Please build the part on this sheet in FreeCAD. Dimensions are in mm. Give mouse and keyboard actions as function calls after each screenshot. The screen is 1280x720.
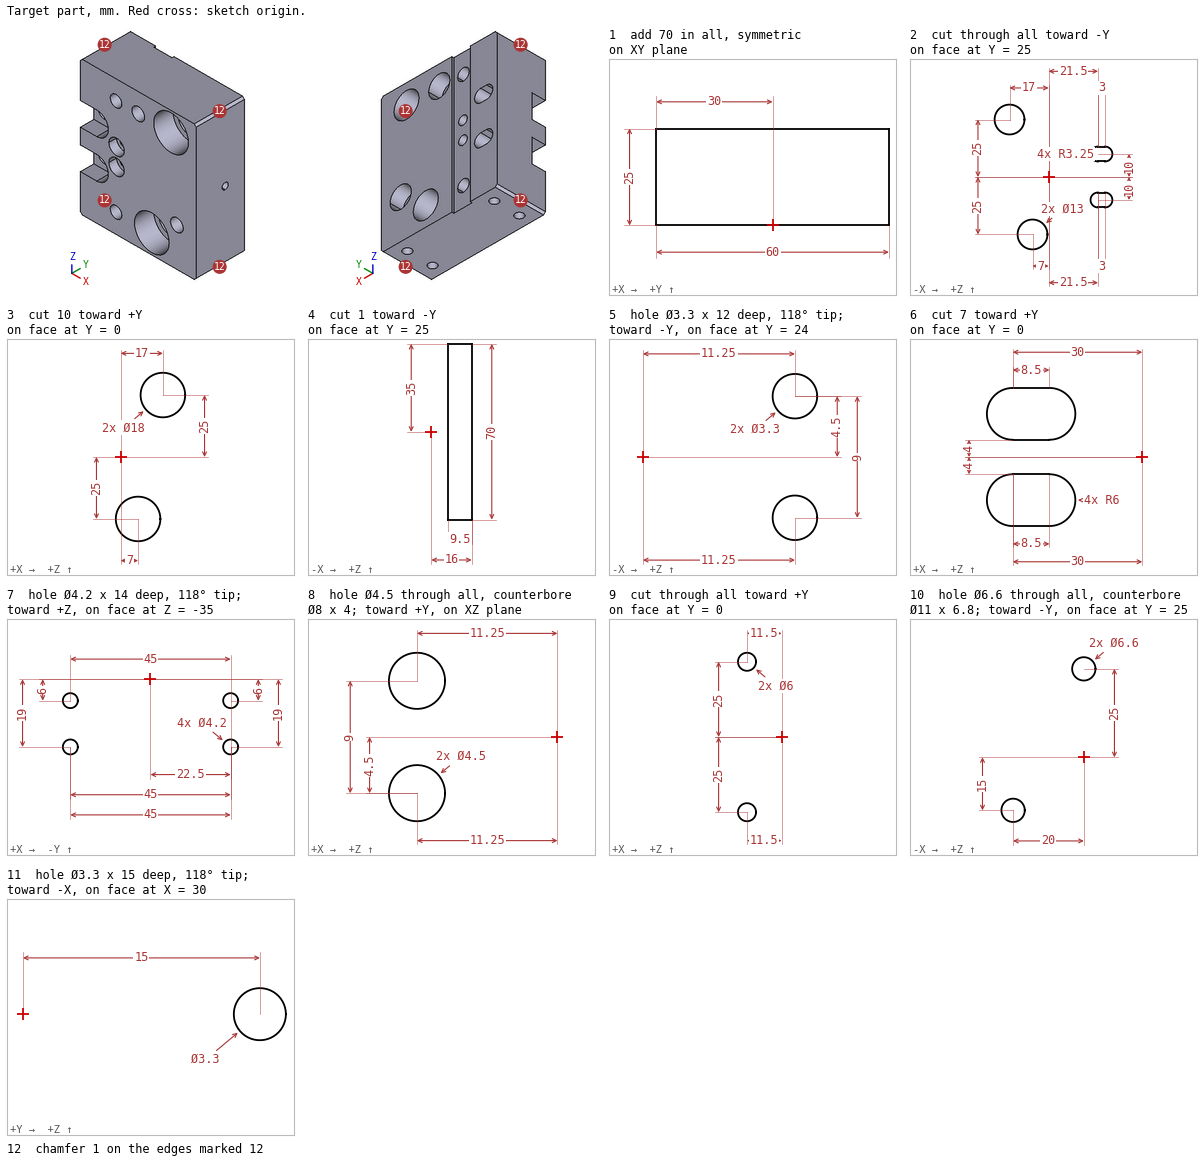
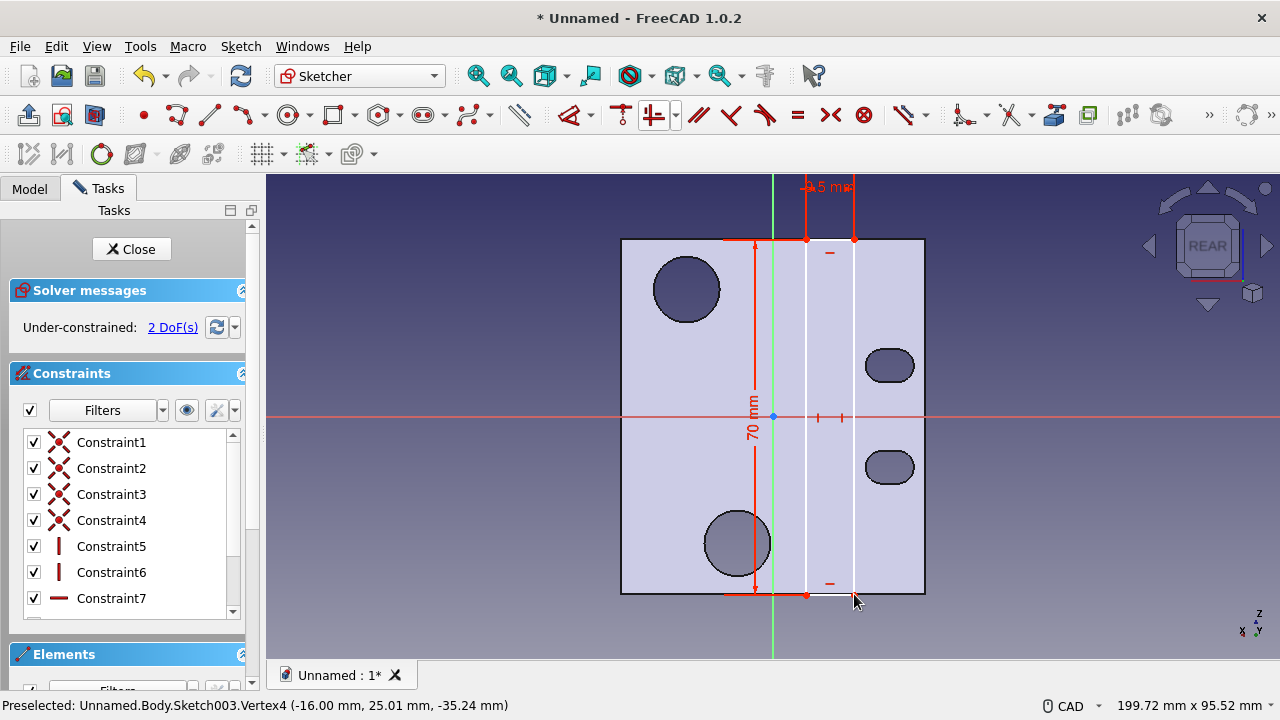
key(d)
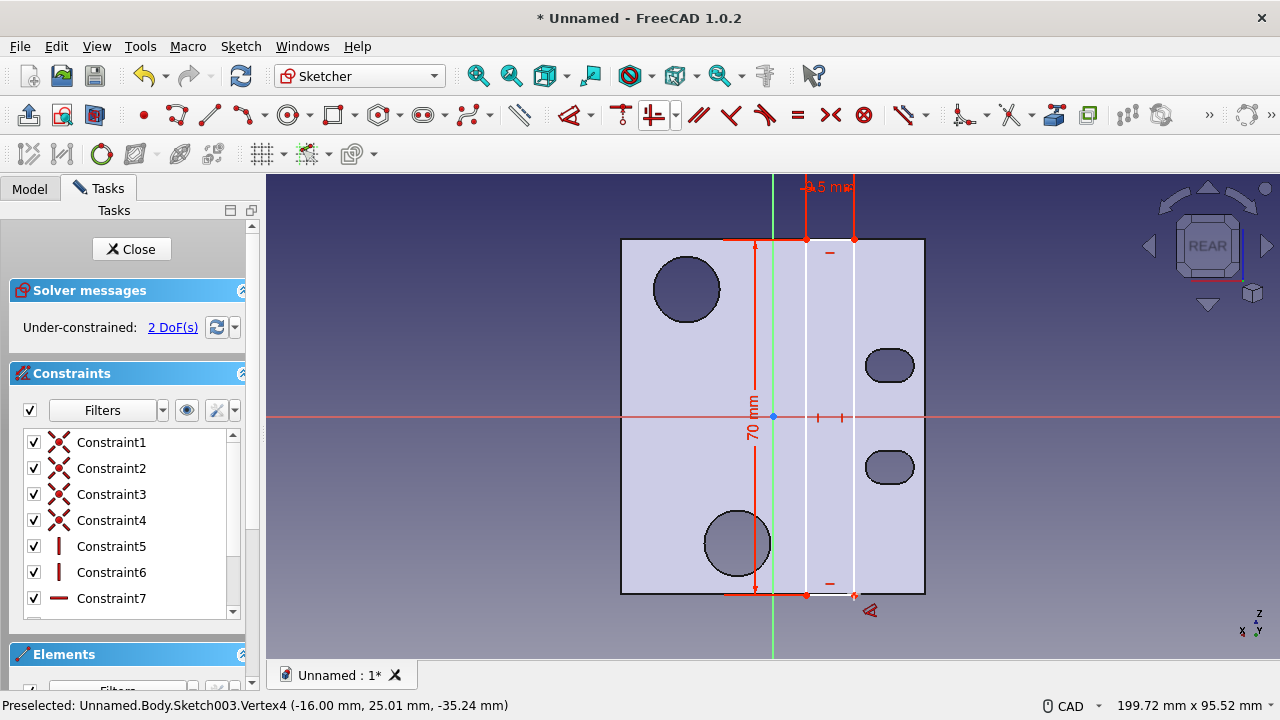
click(806, 240)
click(739, 328)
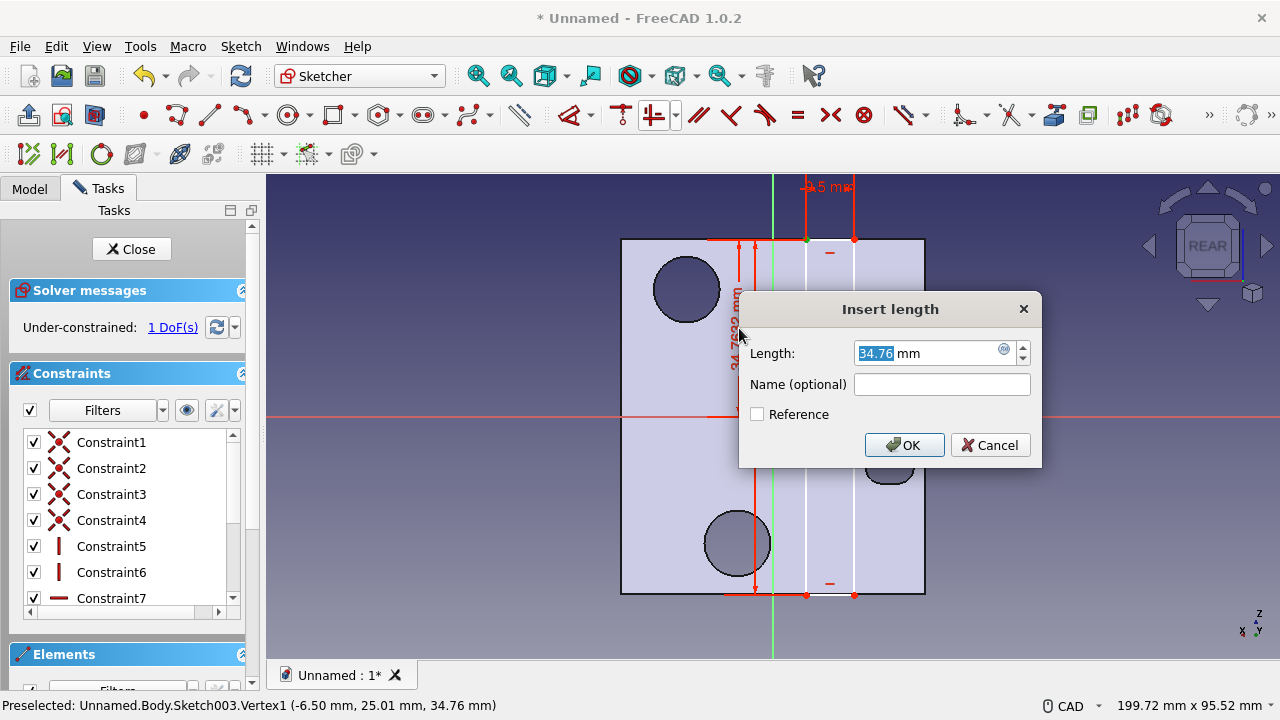
text(35)
key(Return)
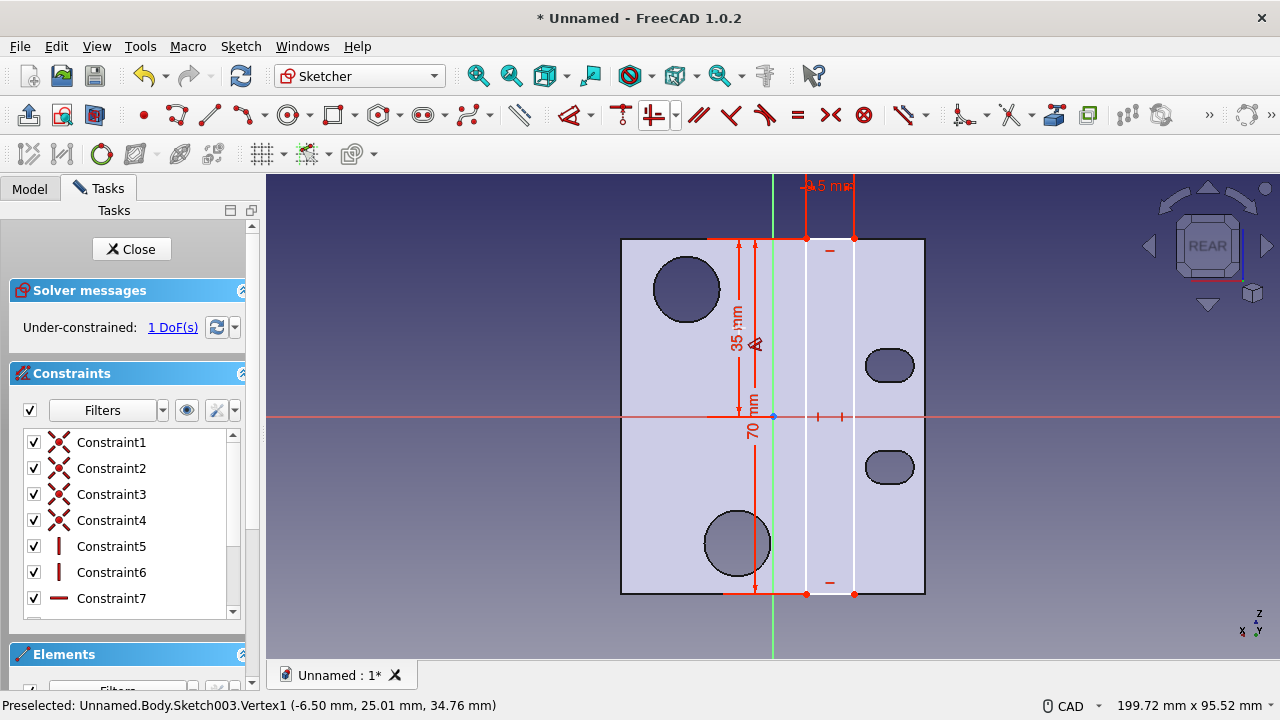
click(854, 594)
click(814, 628)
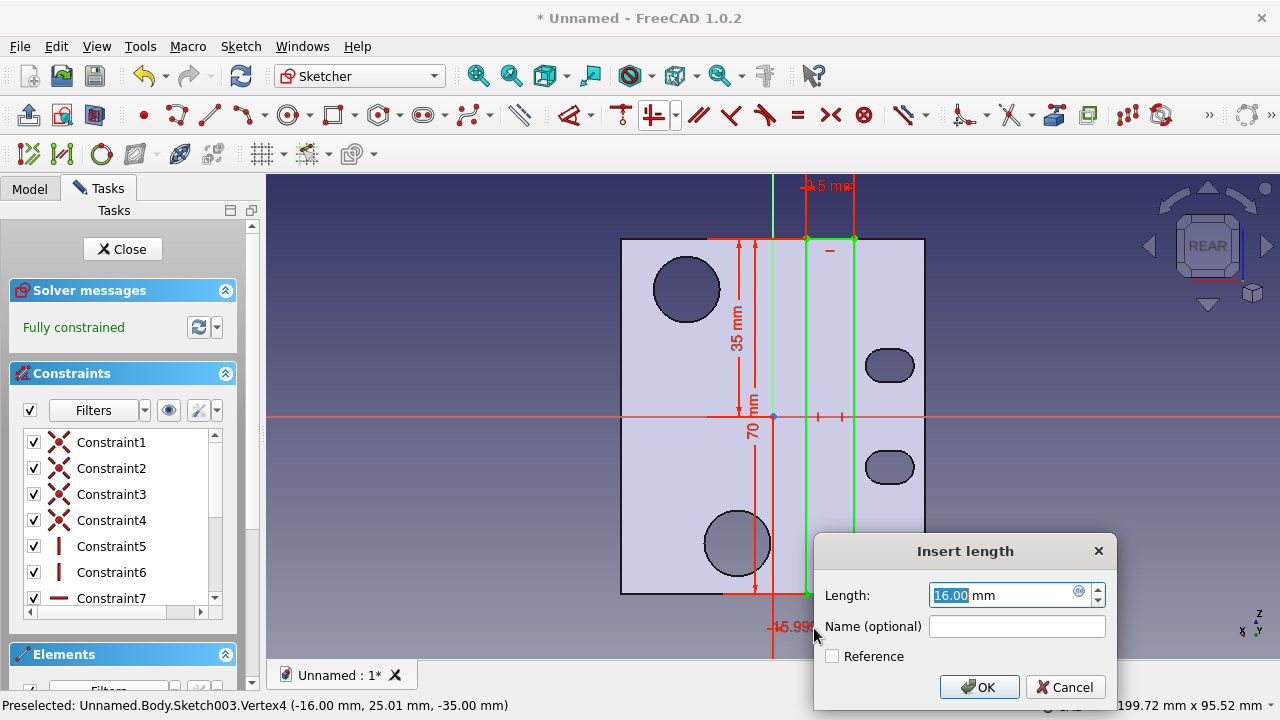
text(16)
key(Return)
key(Escape)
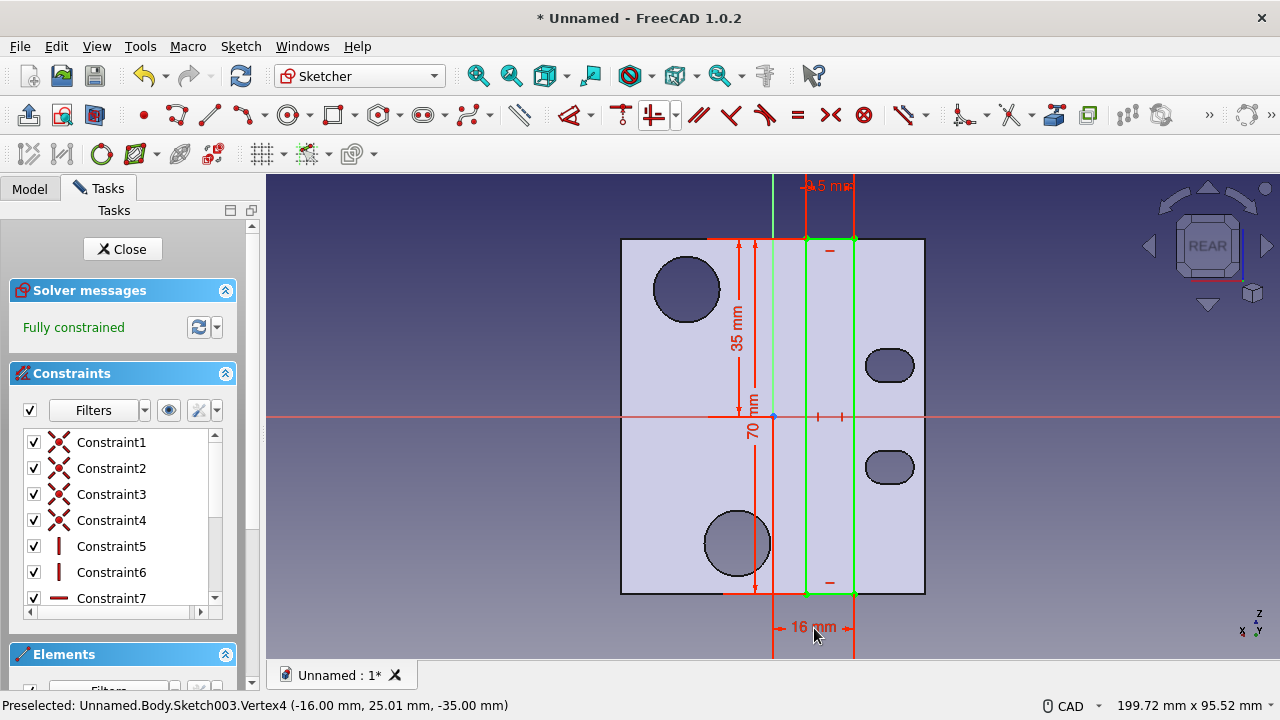
click(123, 249)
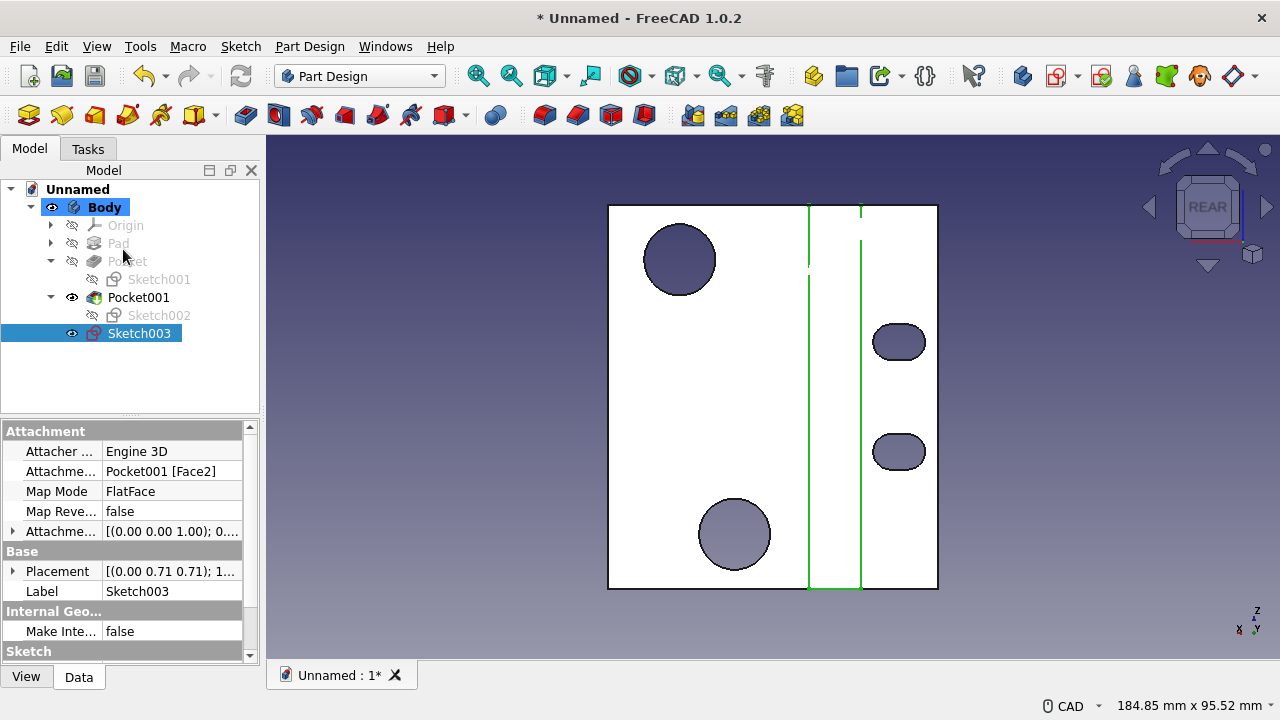
click(246, 116)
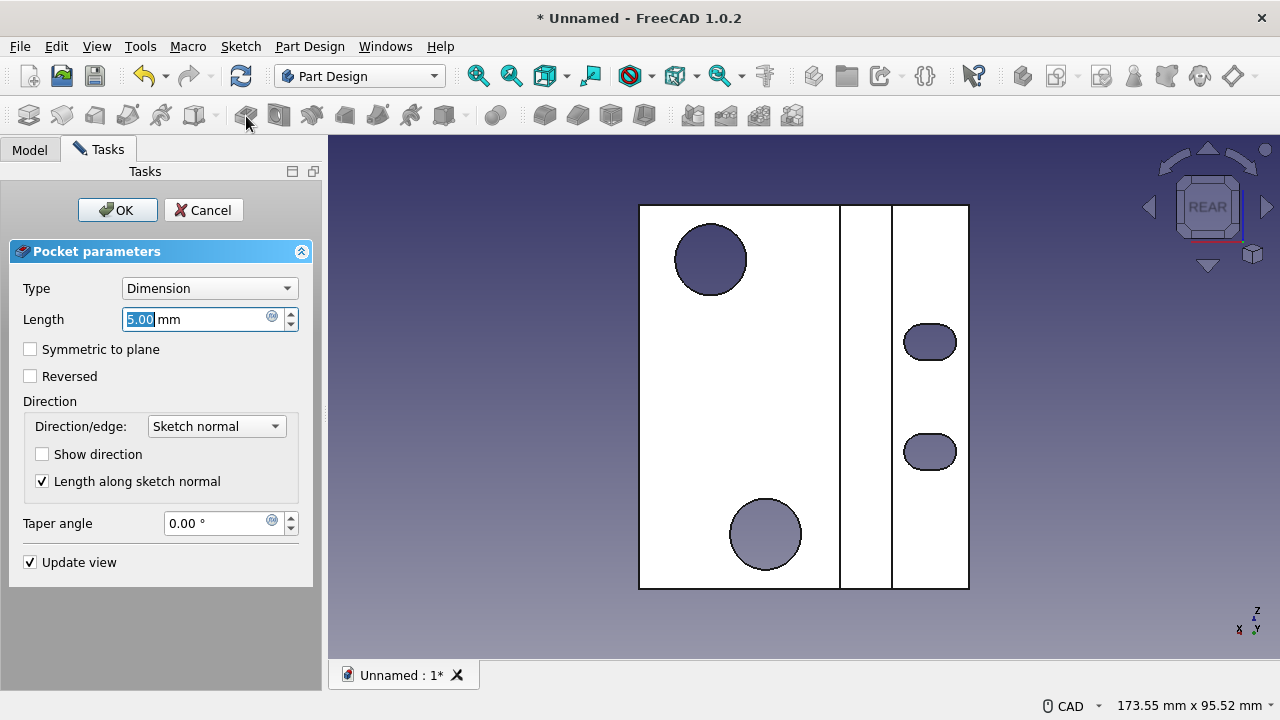
text(1)
key(Tab)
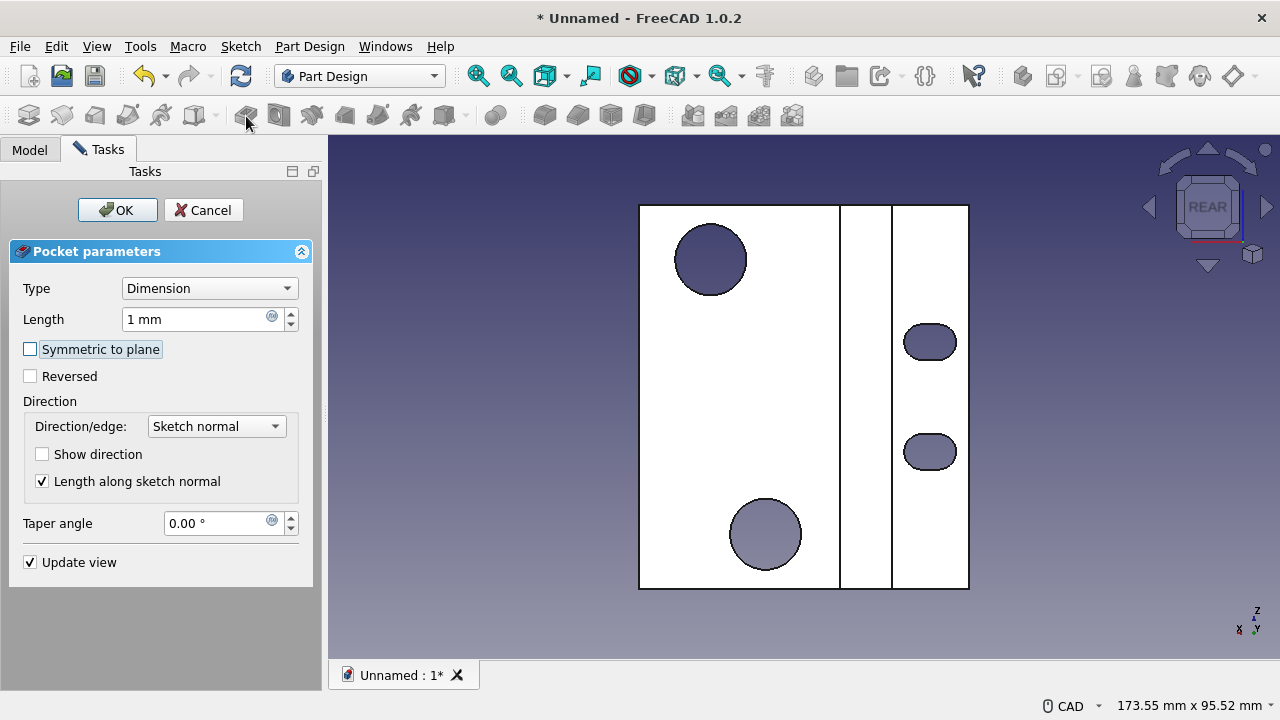
click(118, 210)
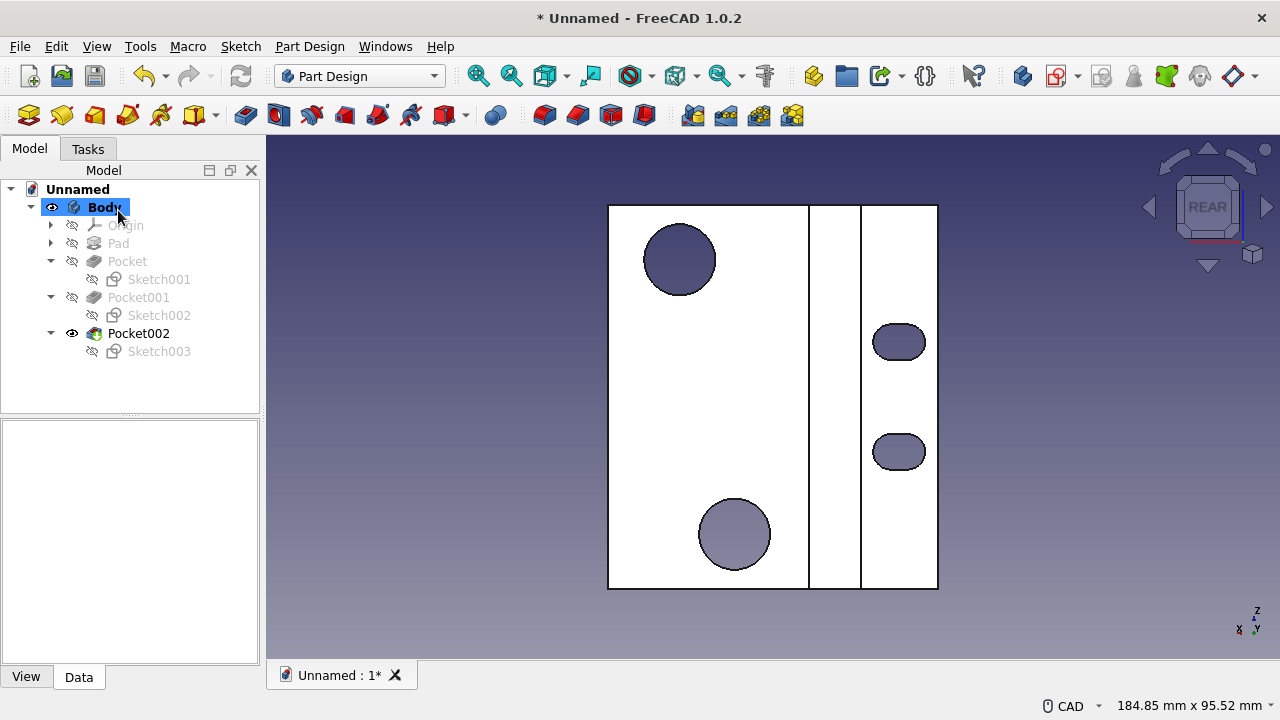
click(835, 231)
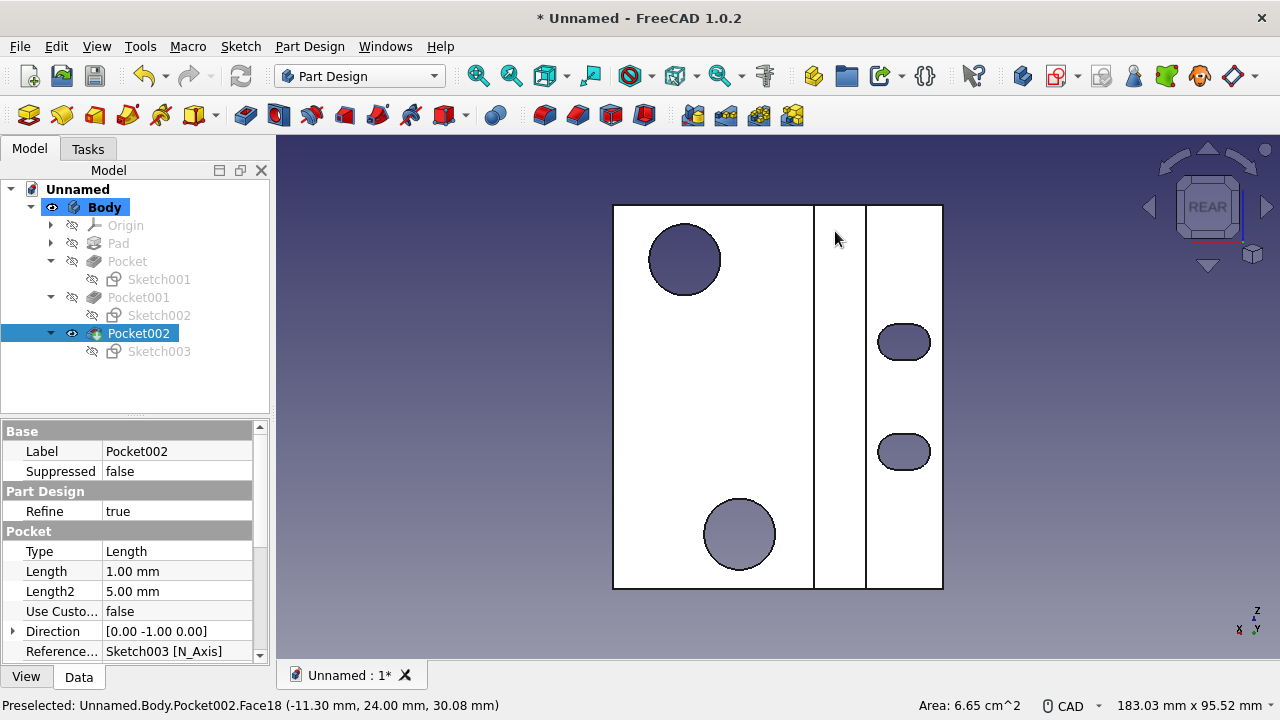
click(1056, 76)